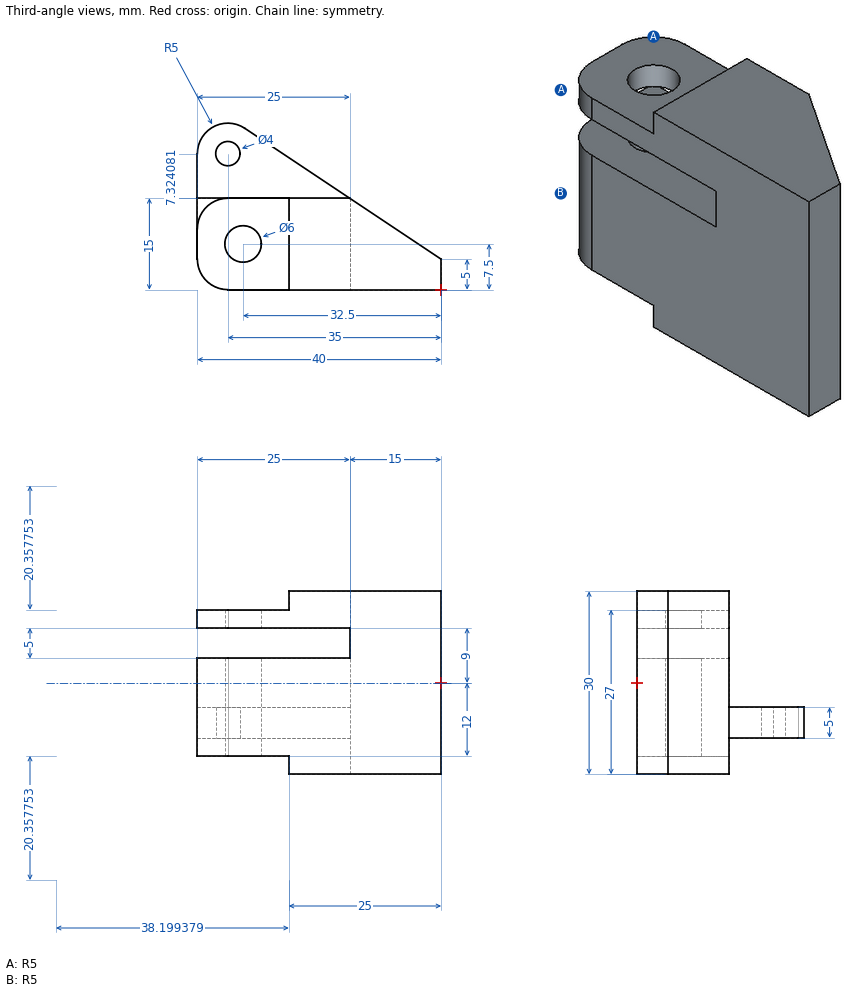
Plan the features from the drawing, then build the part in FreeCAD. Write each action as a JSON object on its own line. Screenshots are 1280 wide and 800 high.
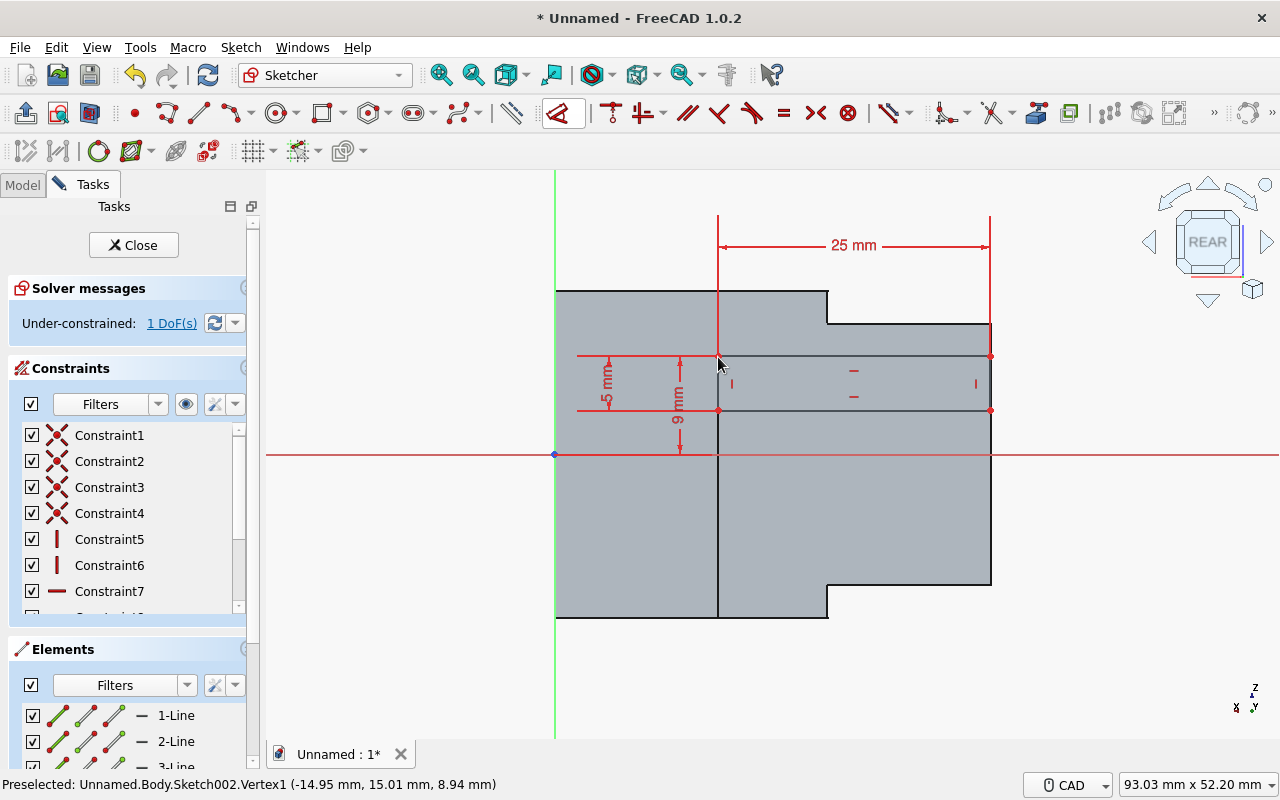
{"action": "left_click", "coordinate": [718, 356]}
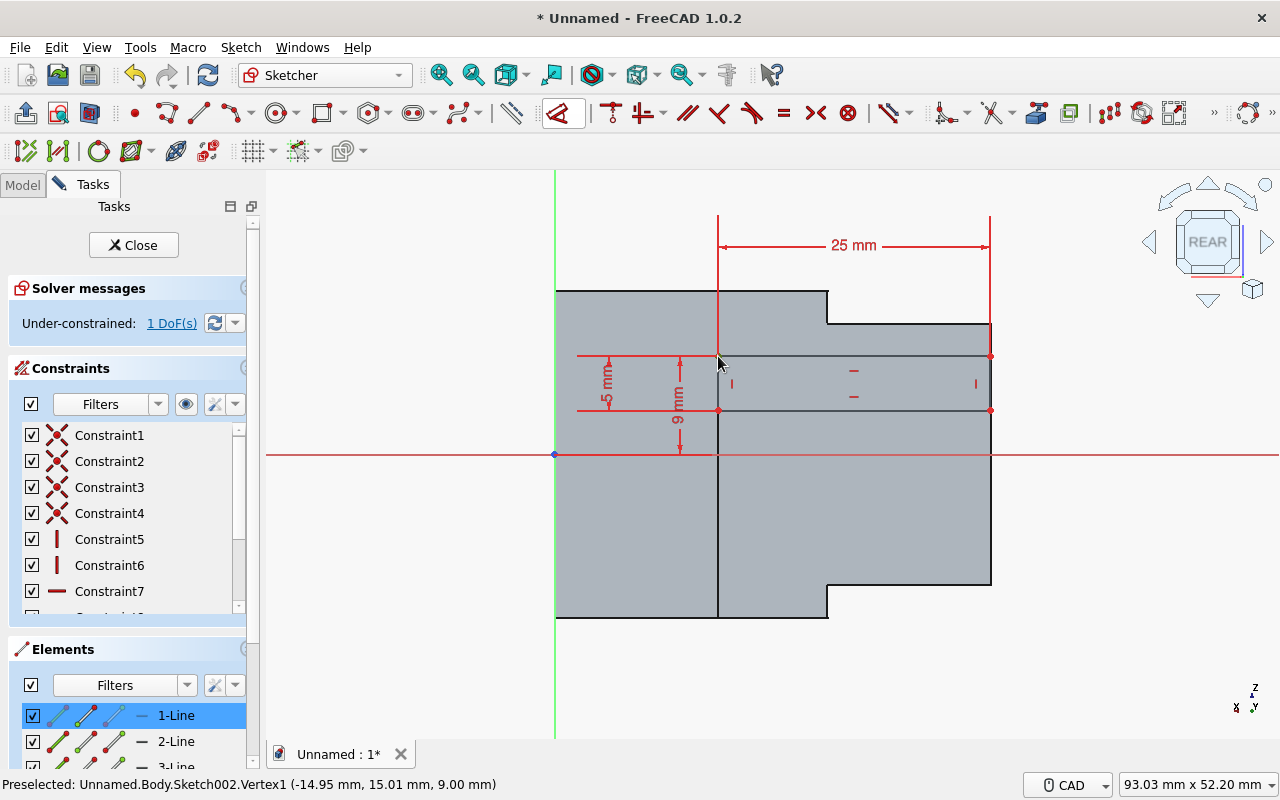
{"action": "key", "text": "l"}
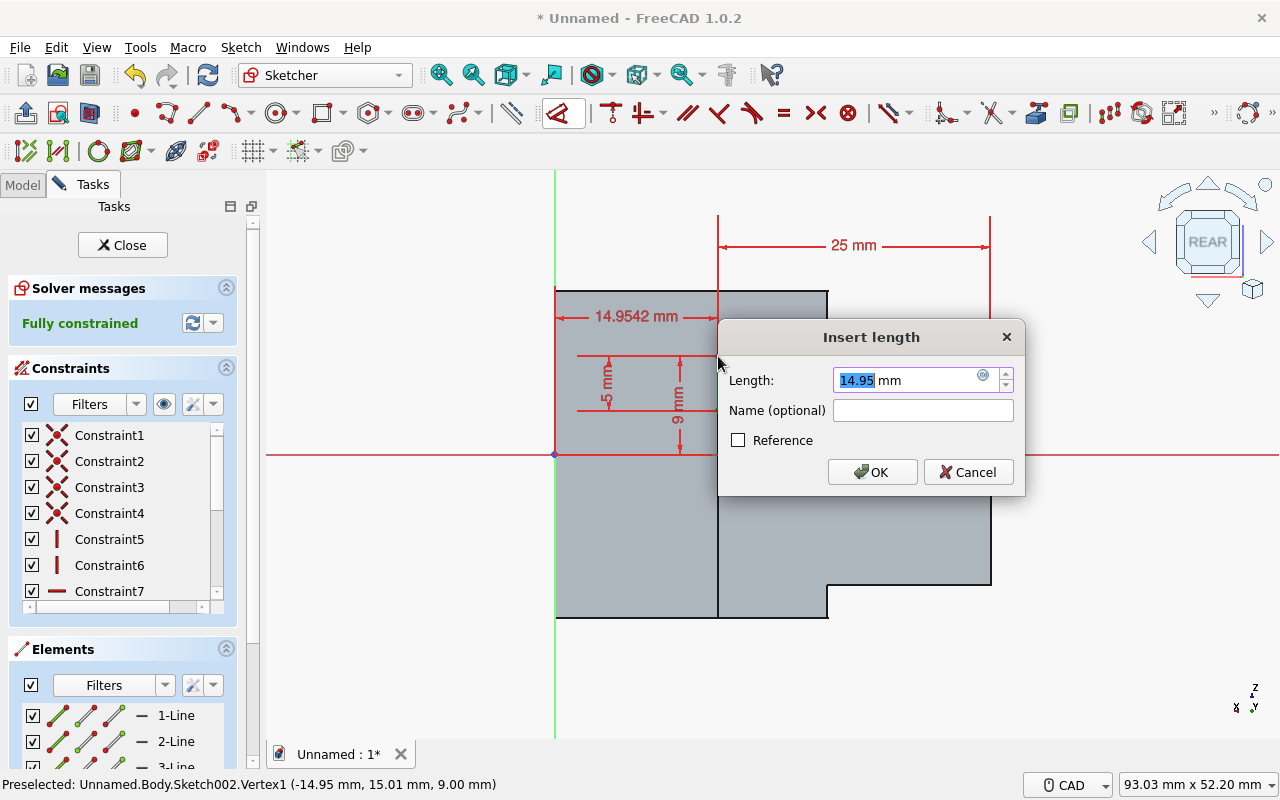
{"action": "type", "text": "15"}
{"action": "key", "text": "Return"}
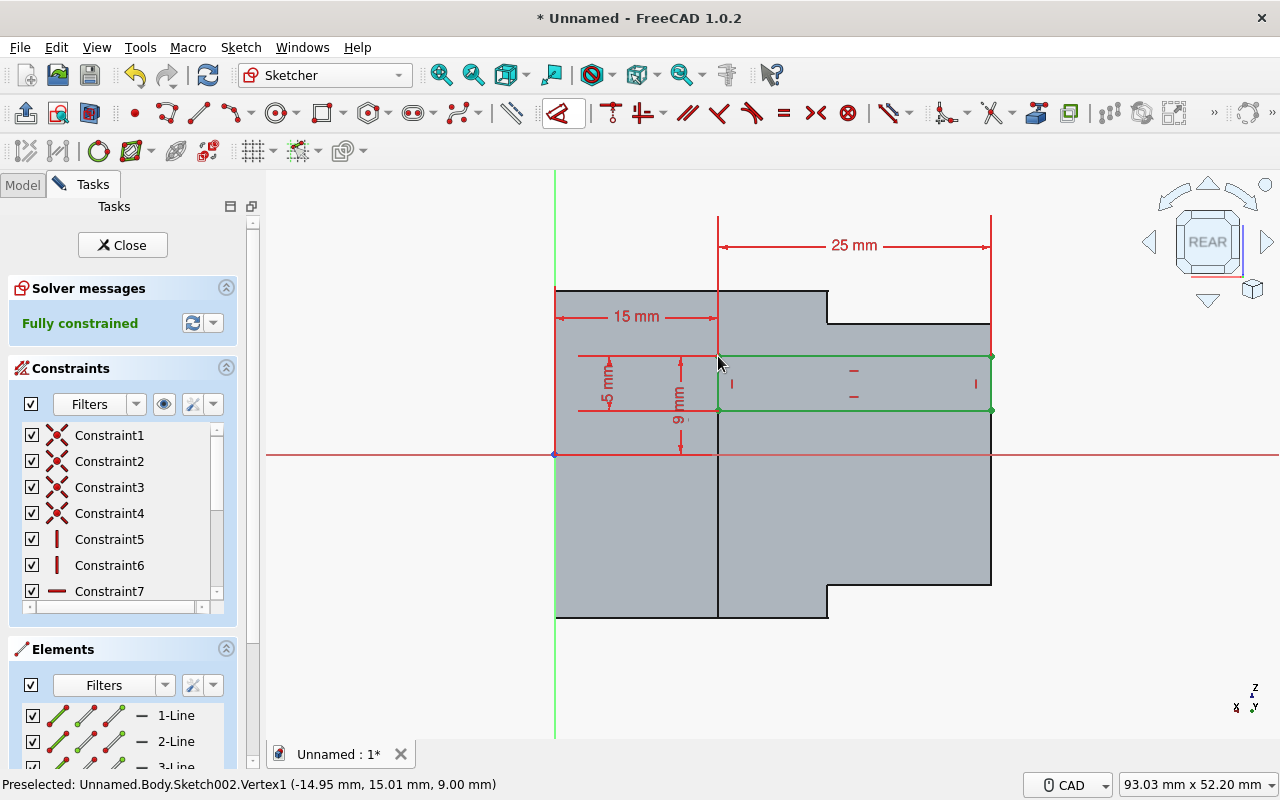
{"action": "left_click", "coordinate": [123, 245]}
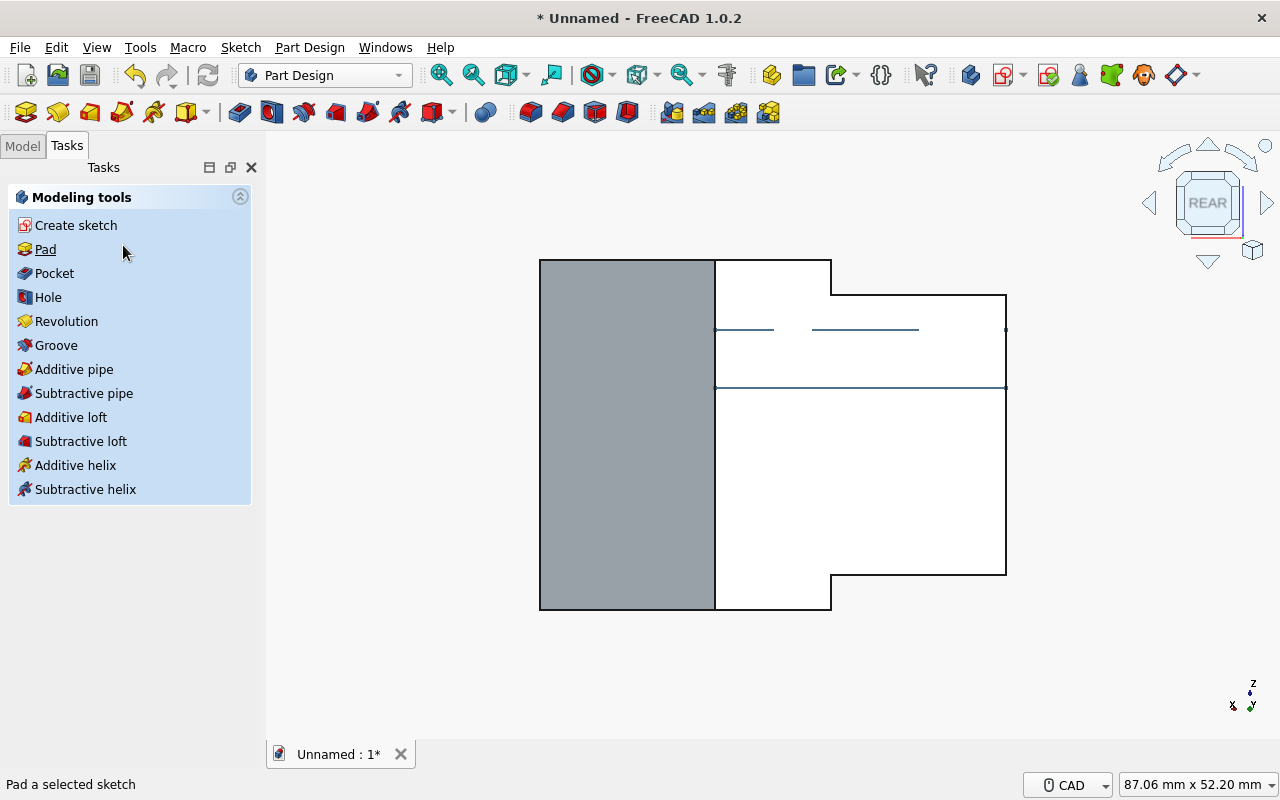
{"action": "left_click", "coordinate": [240, 112]}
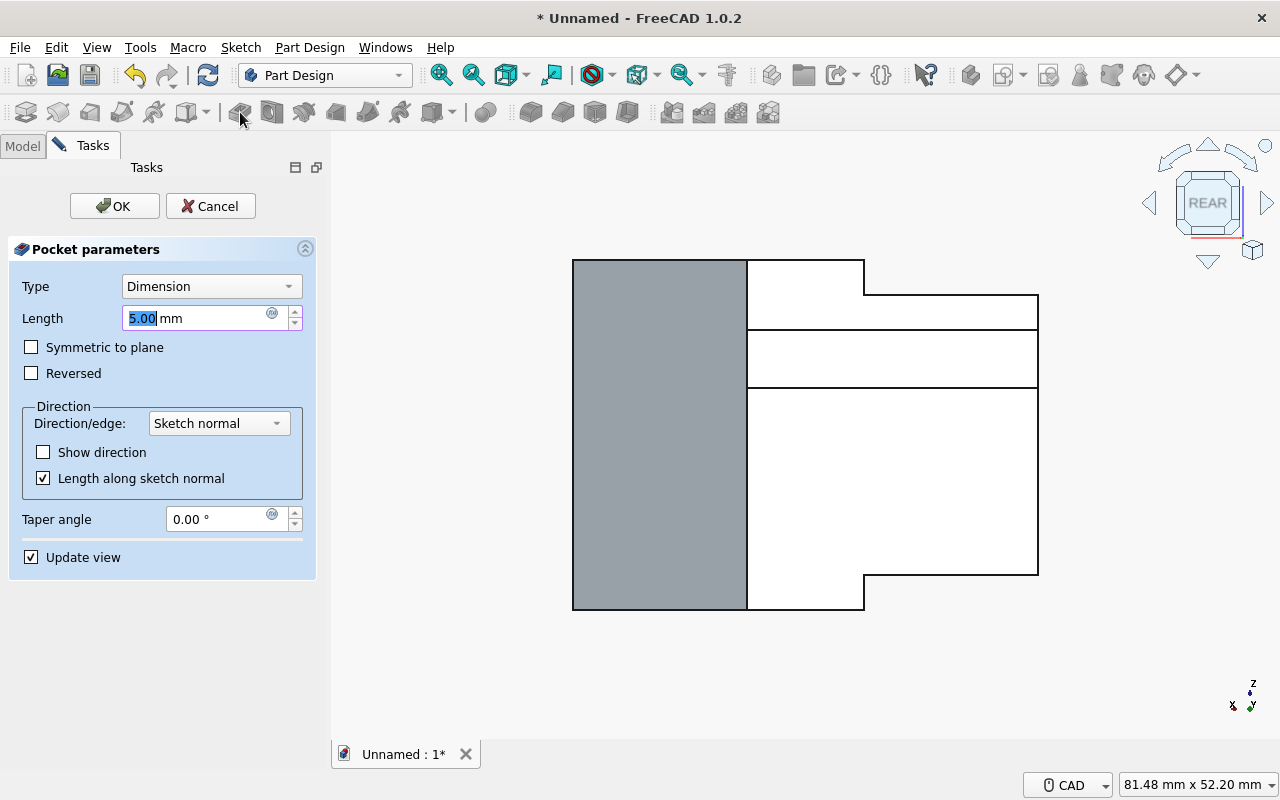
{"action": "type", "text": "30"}
{"action": "key", "text": "Tab"}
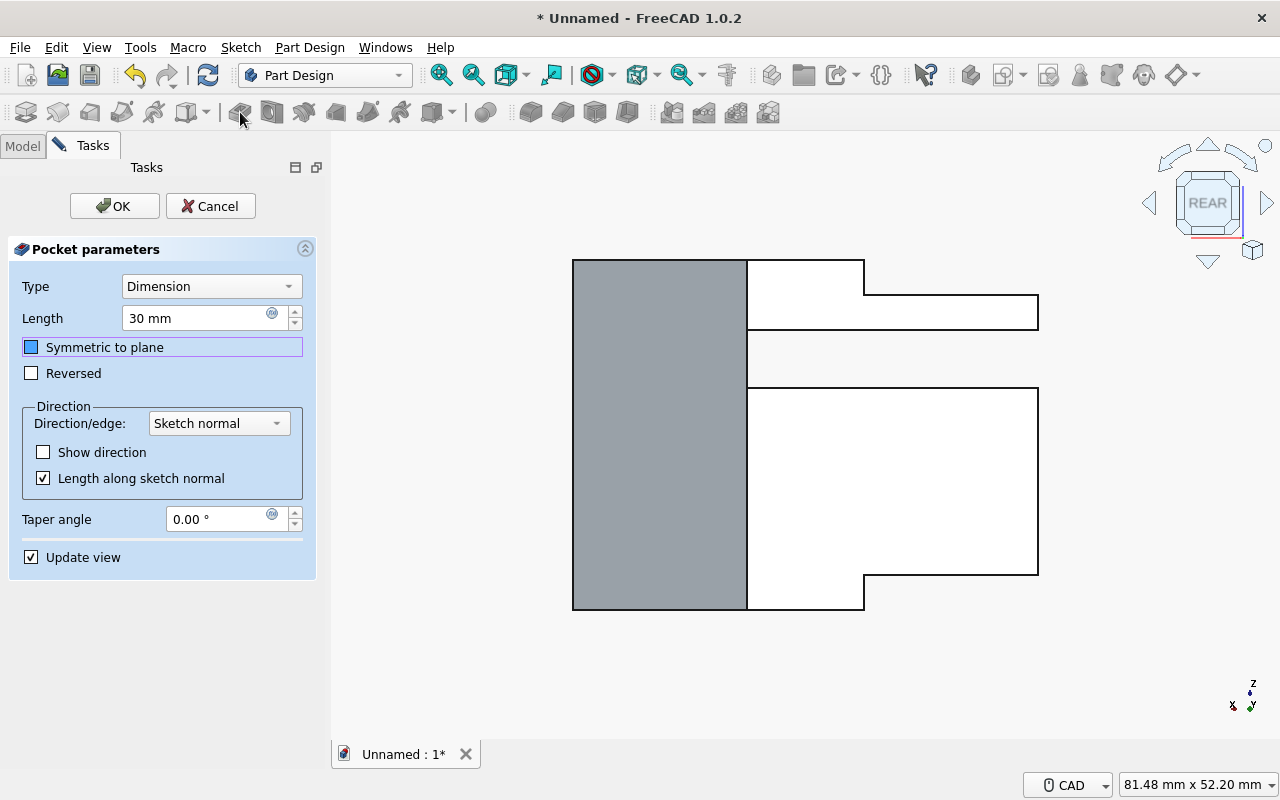
{"action": "left_click", "coordinate": [115, 206]}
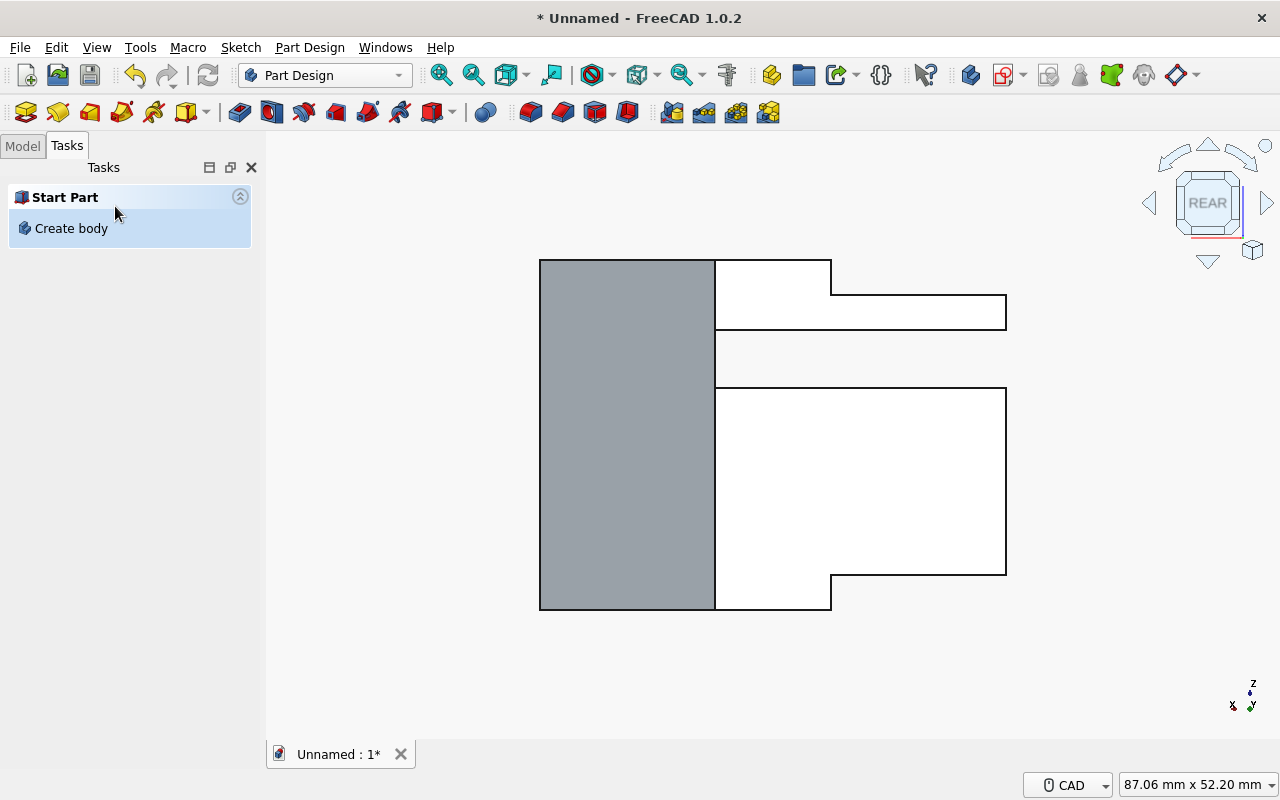
{"action": "left_click", "coordinate": [23, 145]}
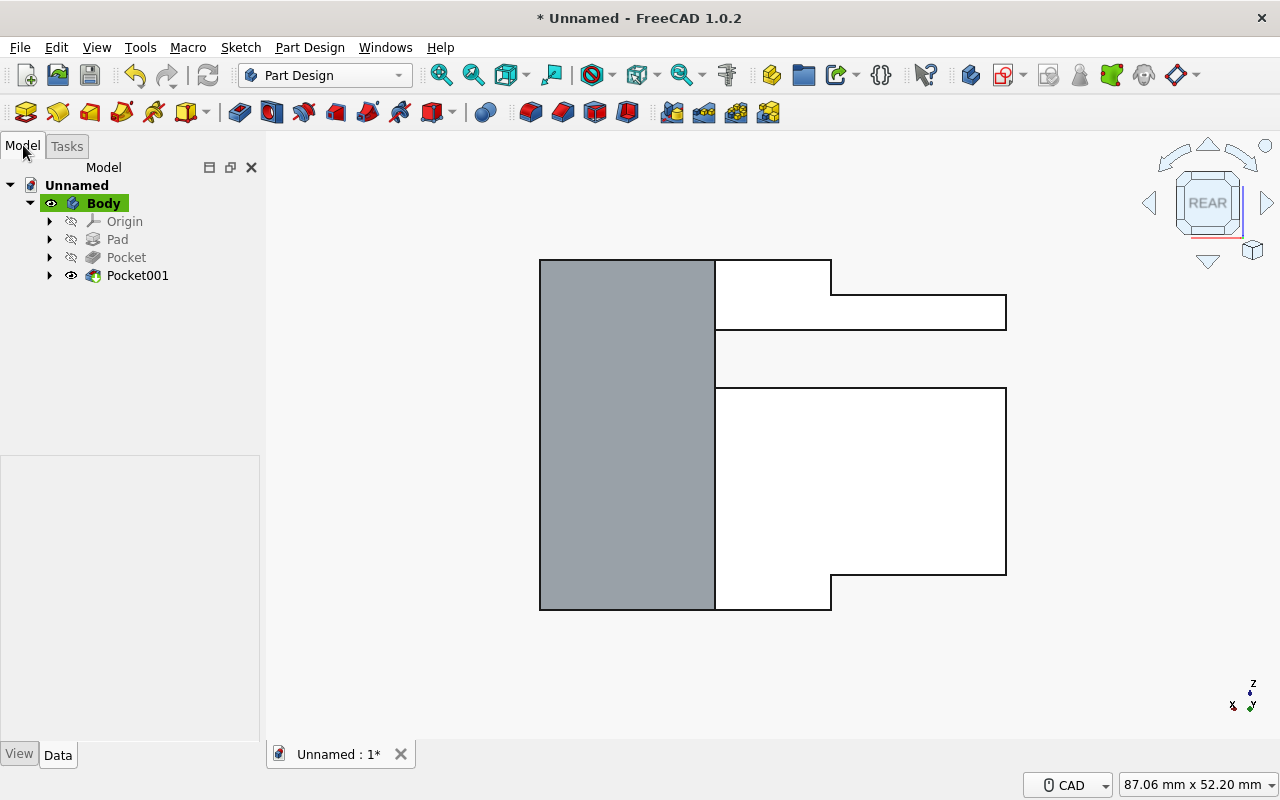
{"action": "left_click", "coordinate": [50, 221]}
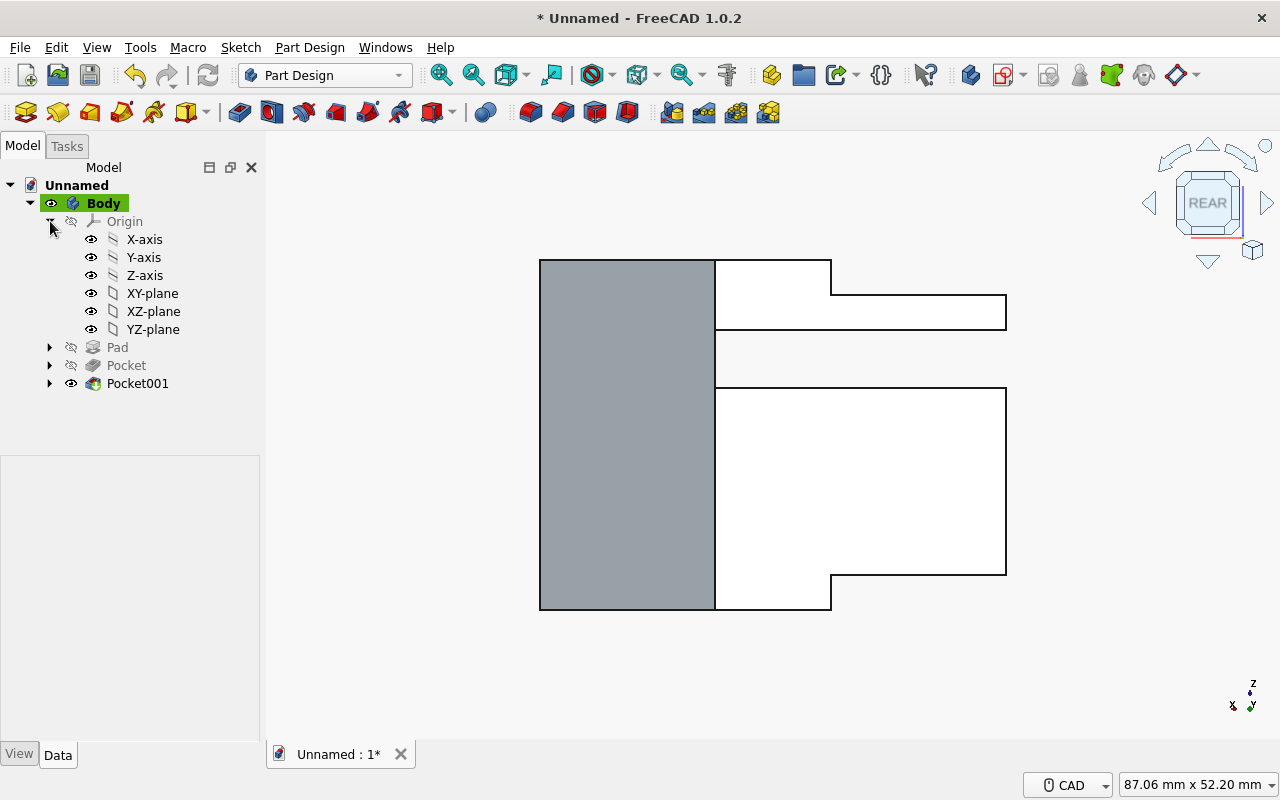
{"action": "left_click", "coordinate": [136, 293]}